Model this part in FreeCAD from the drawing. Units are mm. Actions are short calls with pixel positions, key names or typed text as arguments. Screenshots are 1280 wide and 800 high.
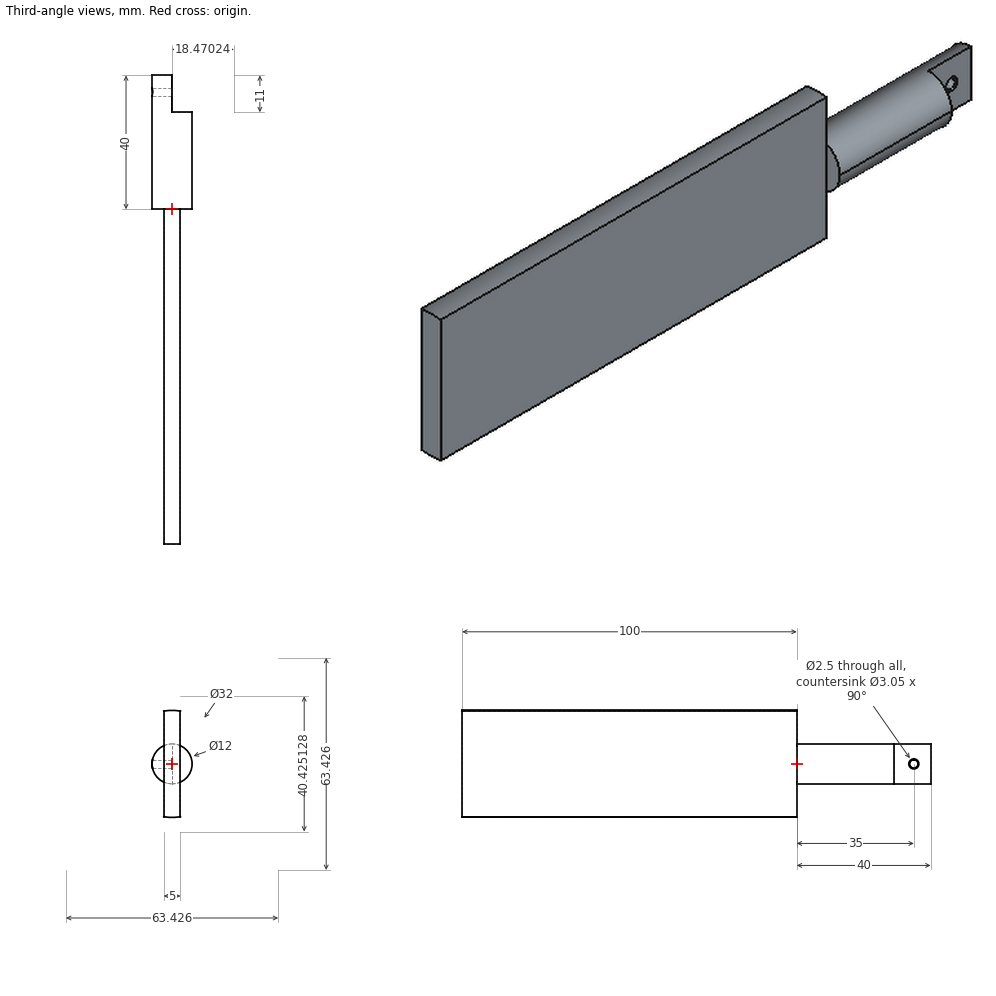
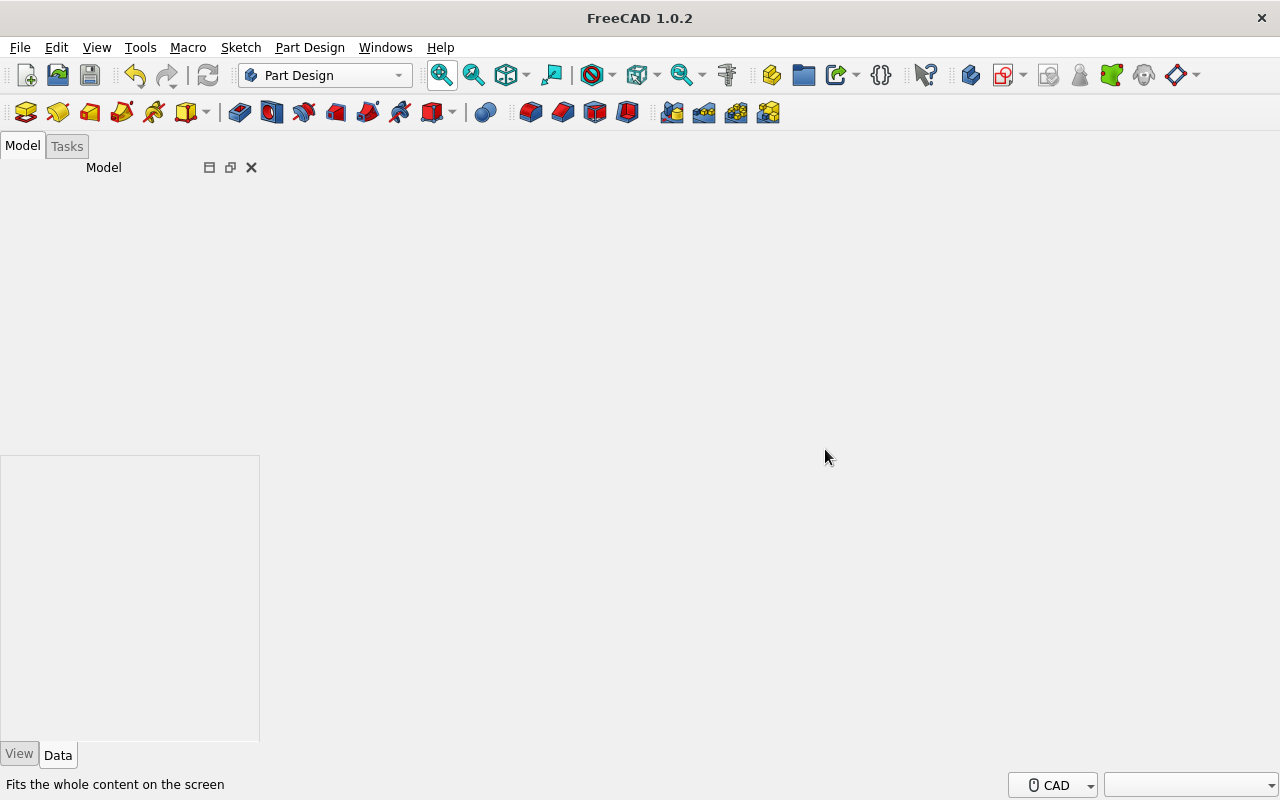
click(26, 76)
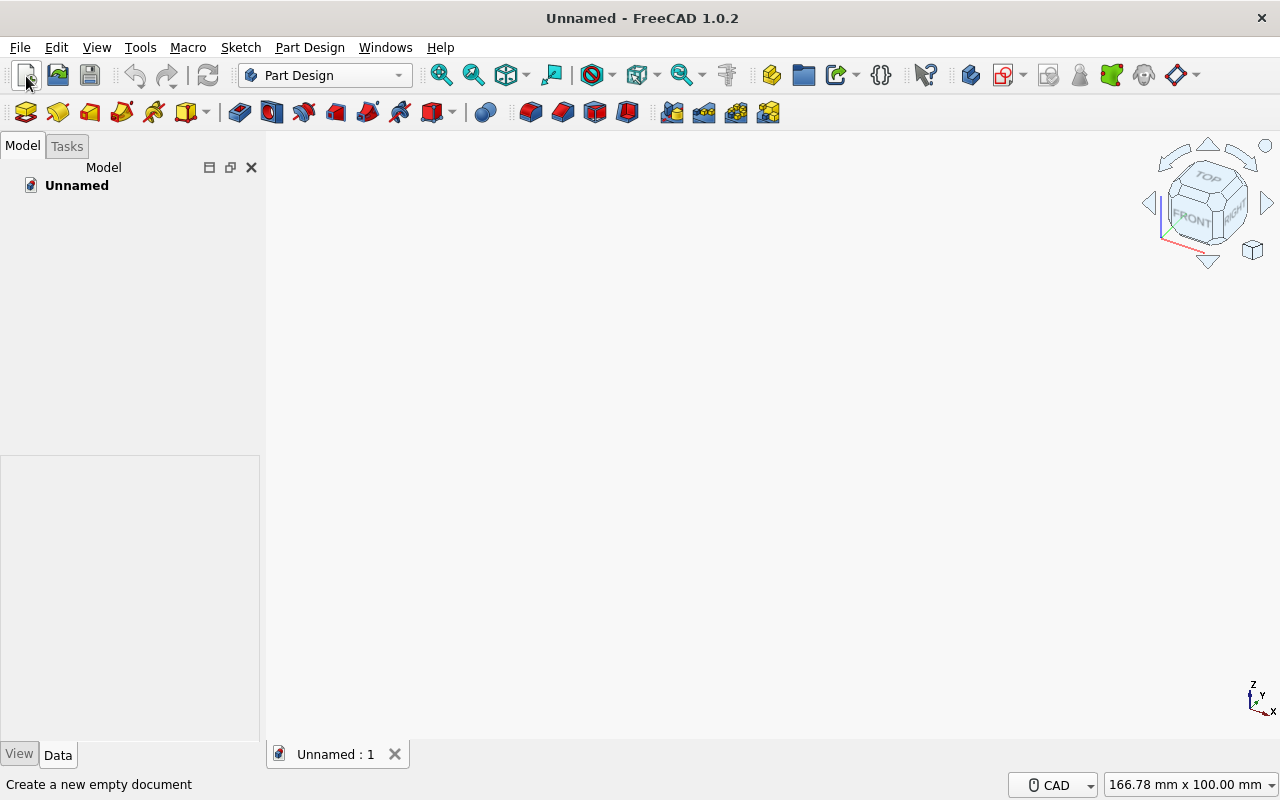
click(1004, 76)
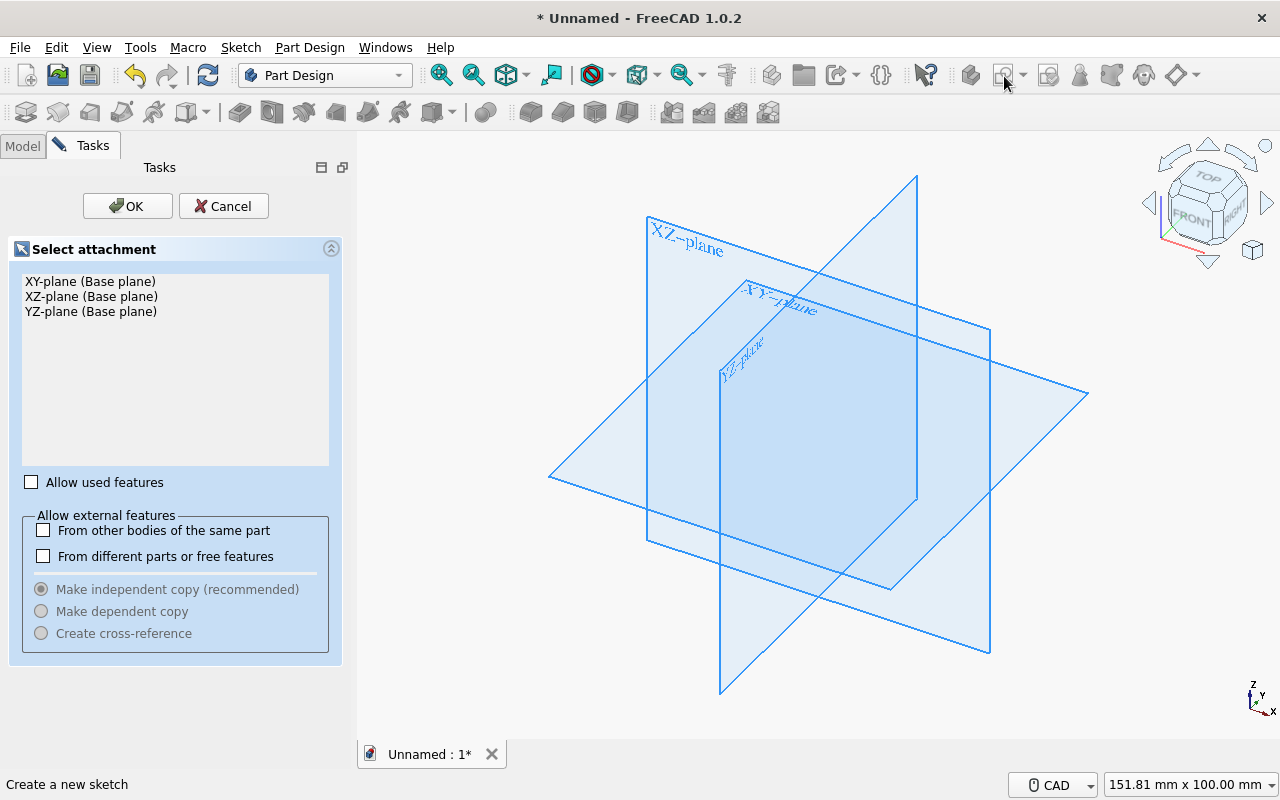
click(82, 296)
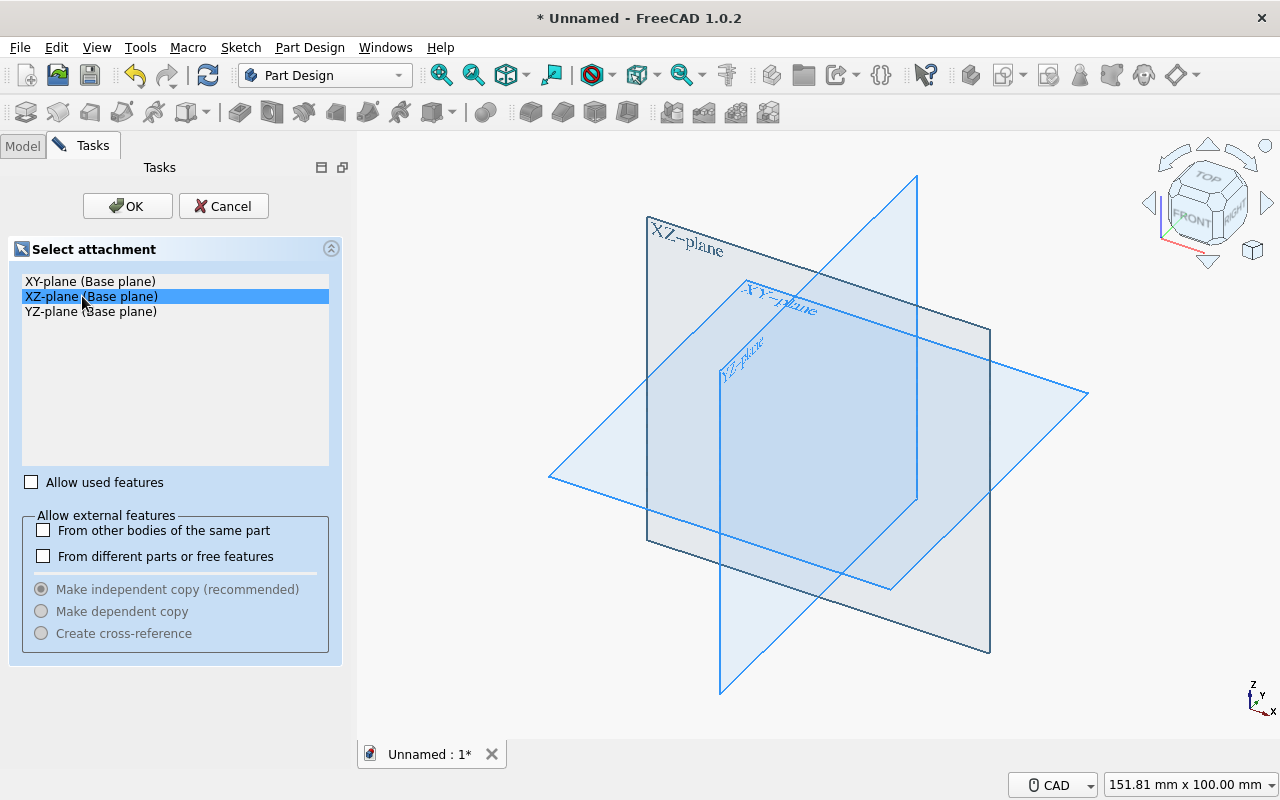
click(128, 206)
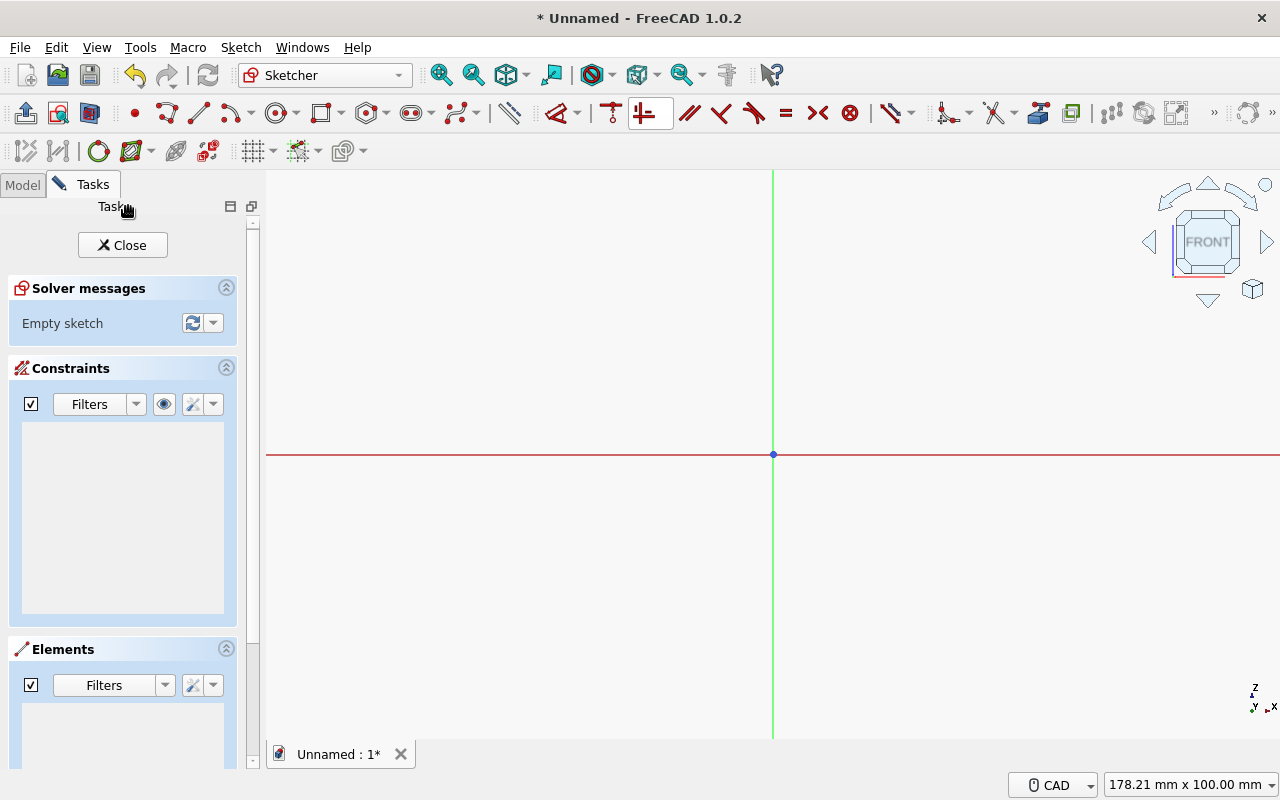
scroll(790, 454, up, 8)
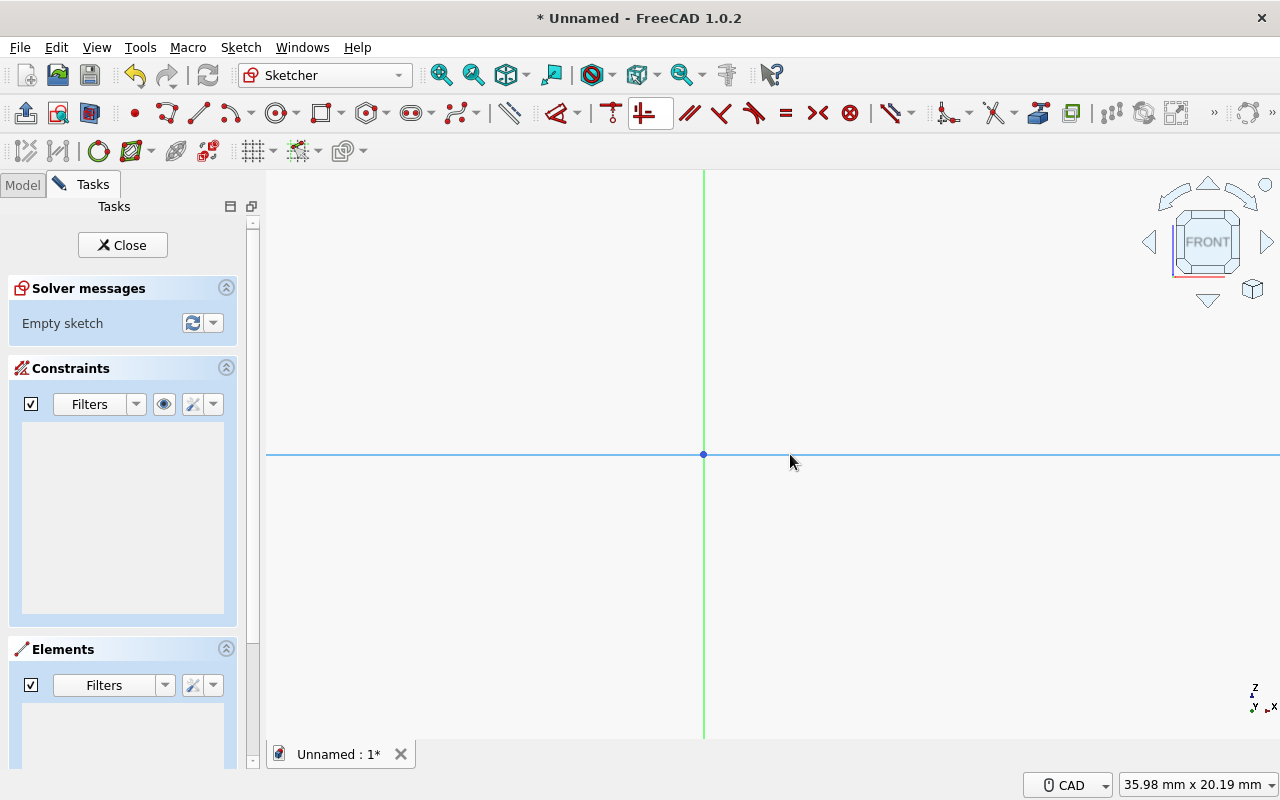
click(276, 114)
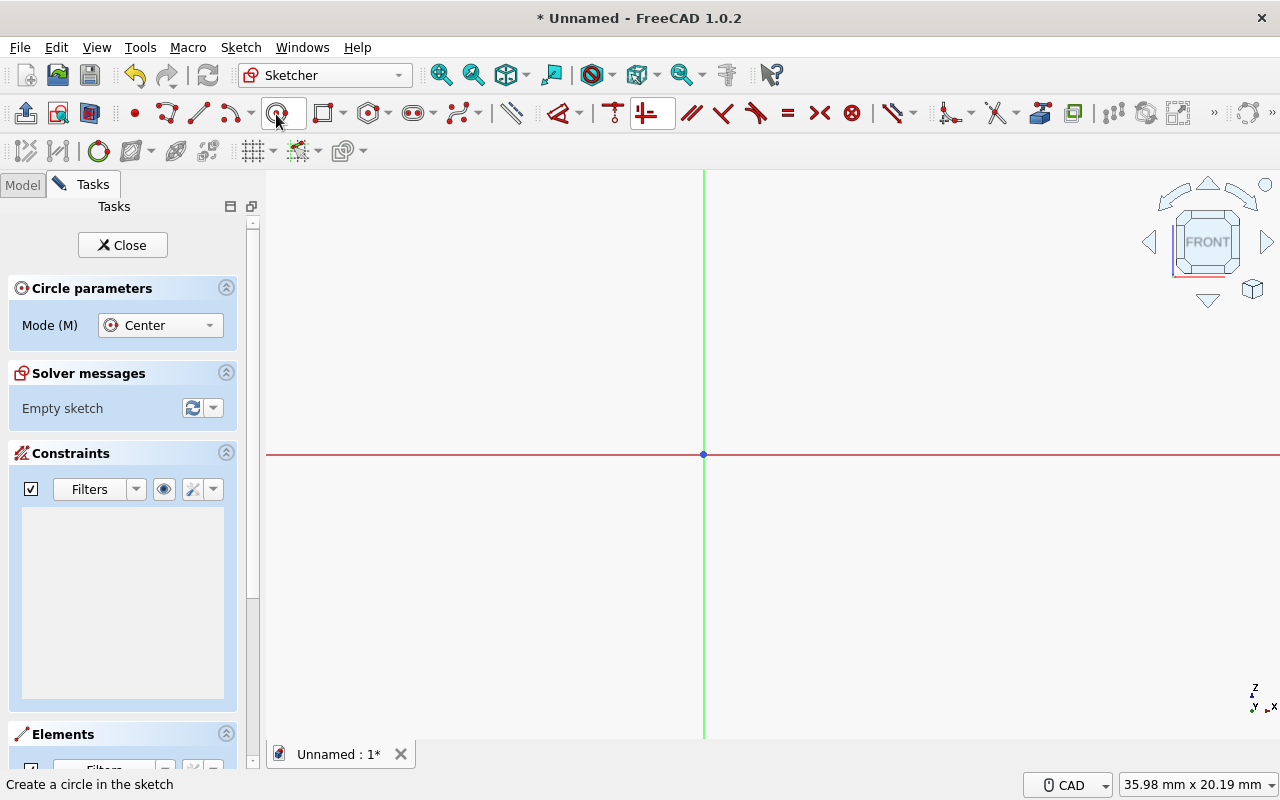
click(704, 454)
move(823, 335)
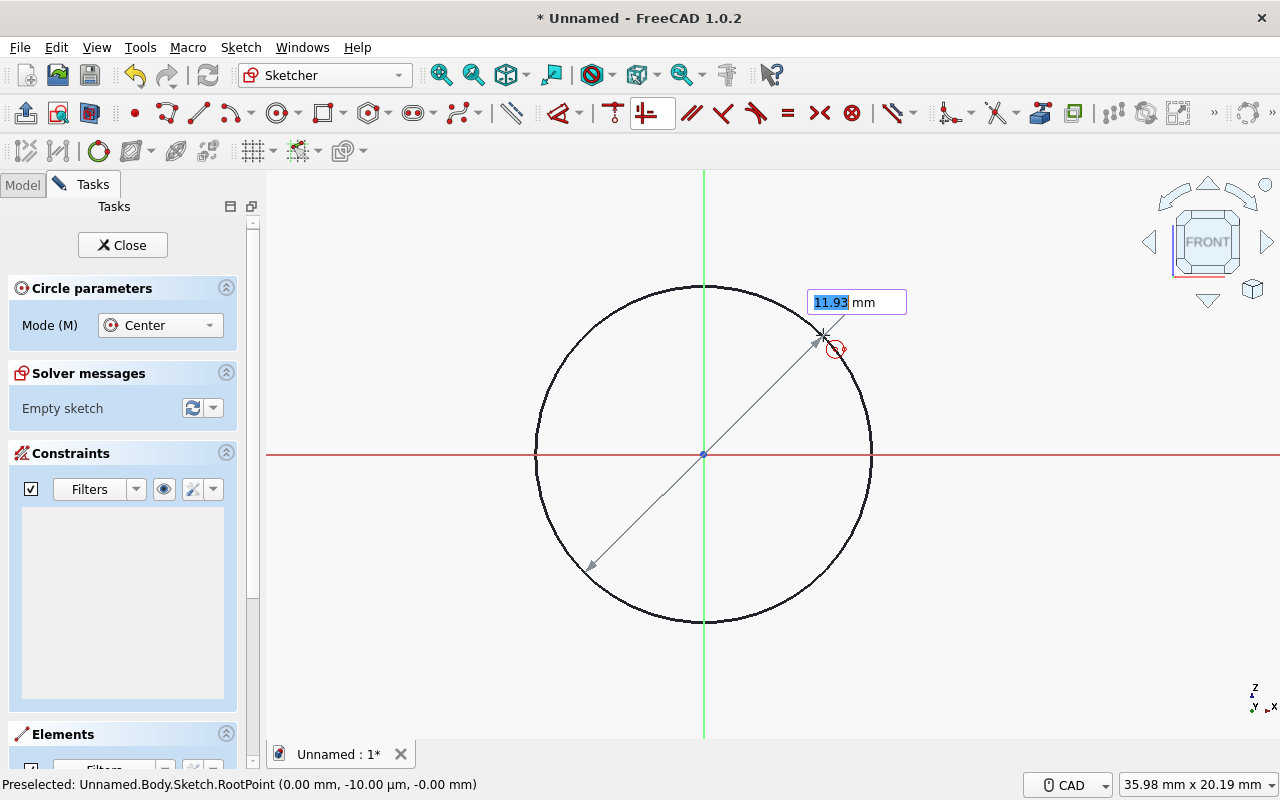
text(12)
key(Return)
key(Escape)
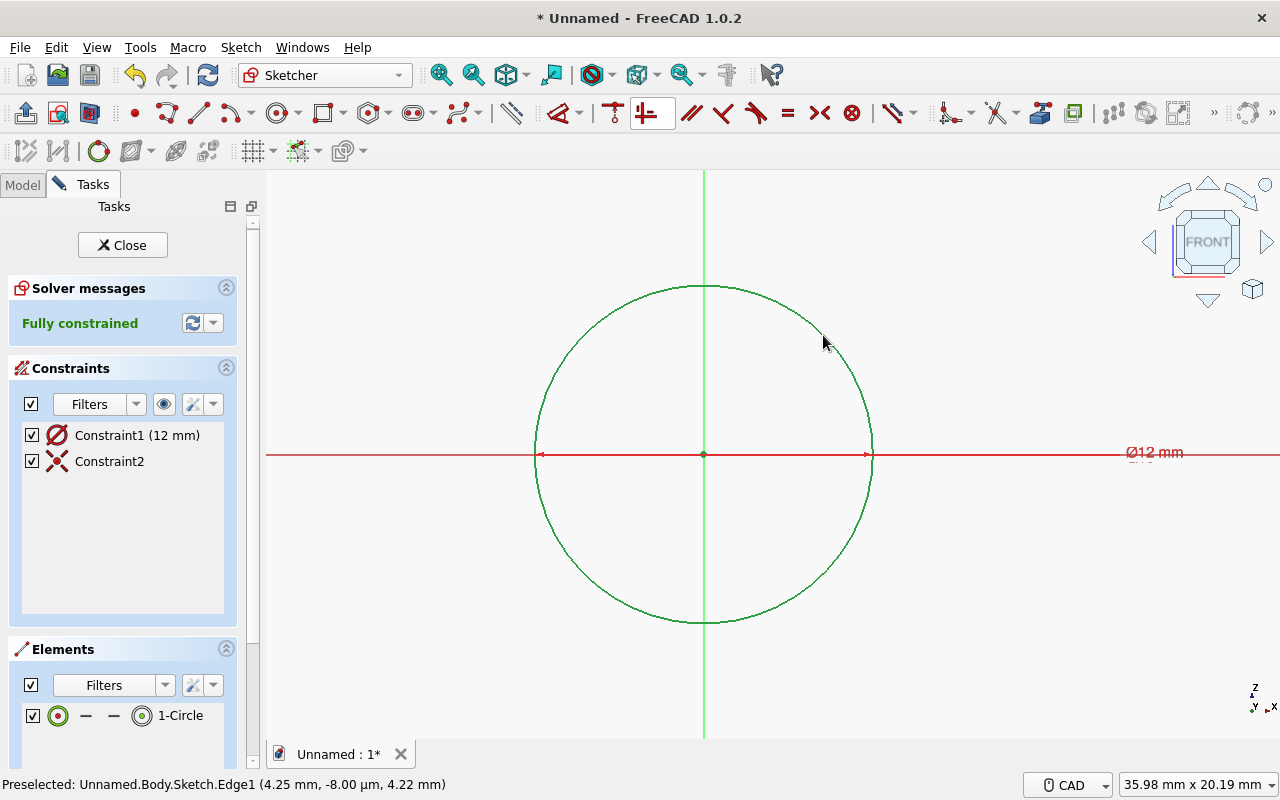
click(123, 245)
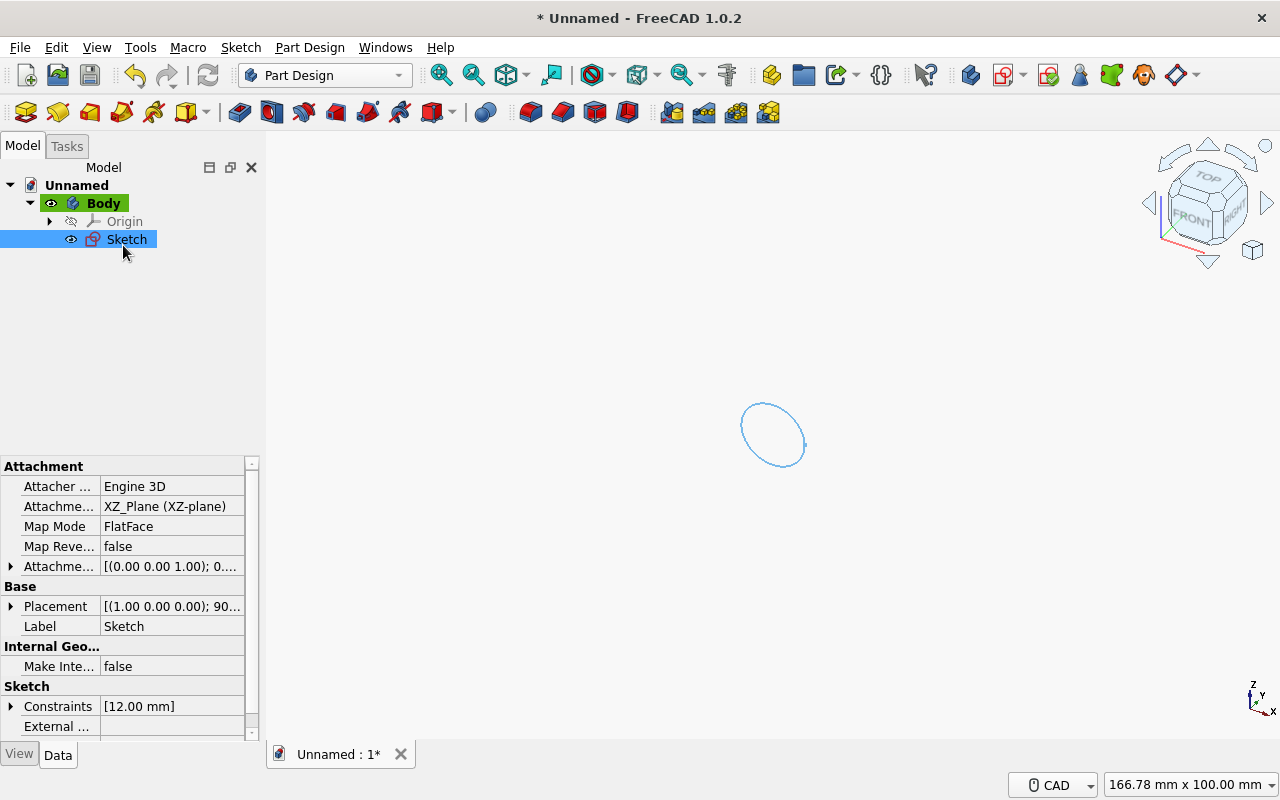
click(26, 112)